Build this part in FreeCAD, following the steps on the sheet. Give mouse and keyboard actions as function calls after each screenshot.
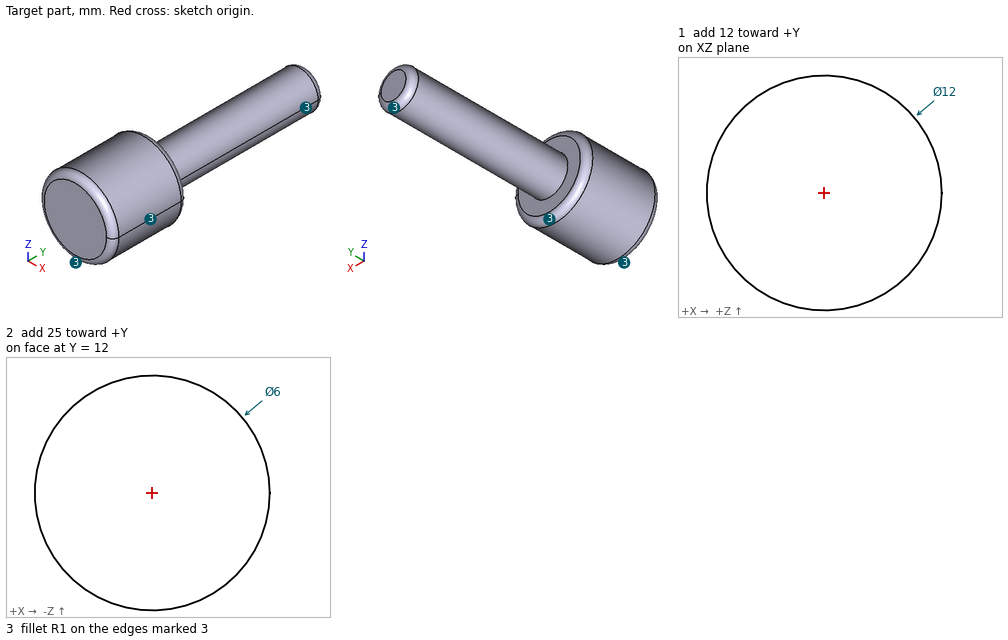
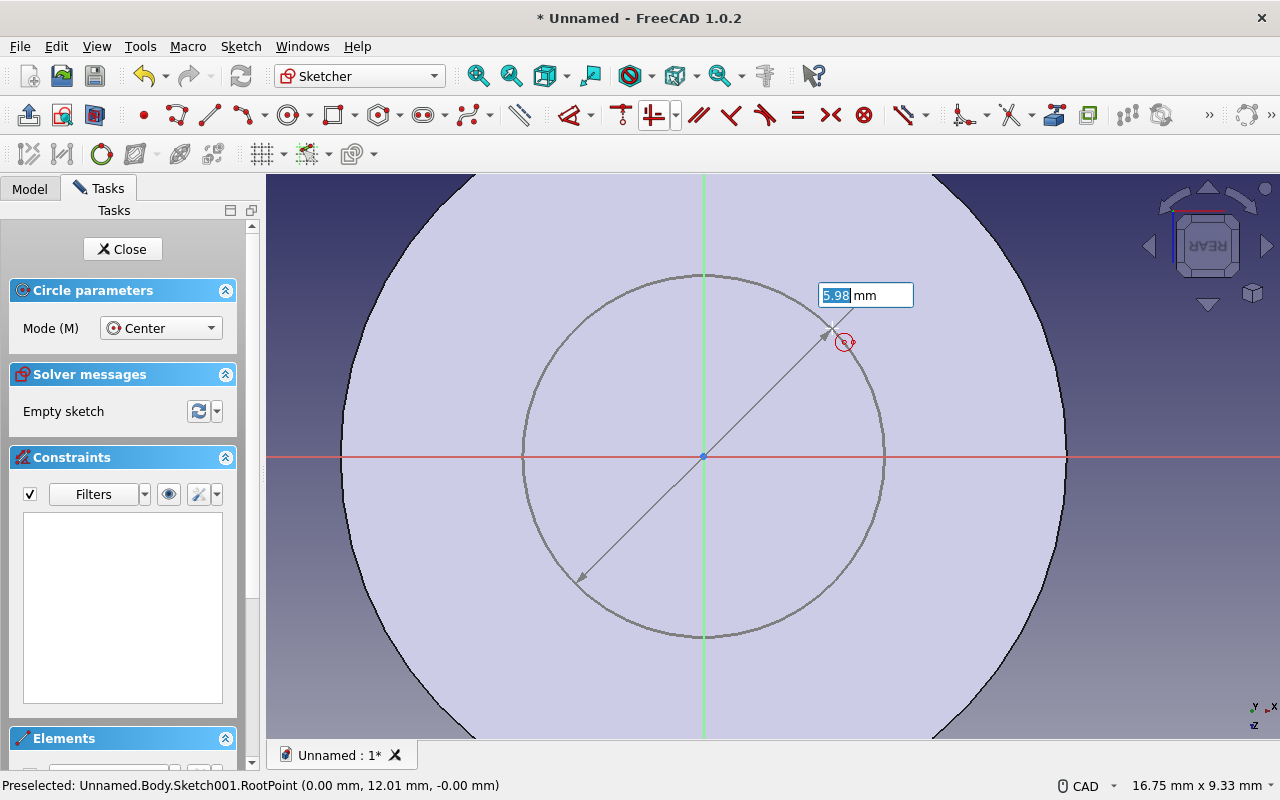
text(6)
key(Return)
key(Escape)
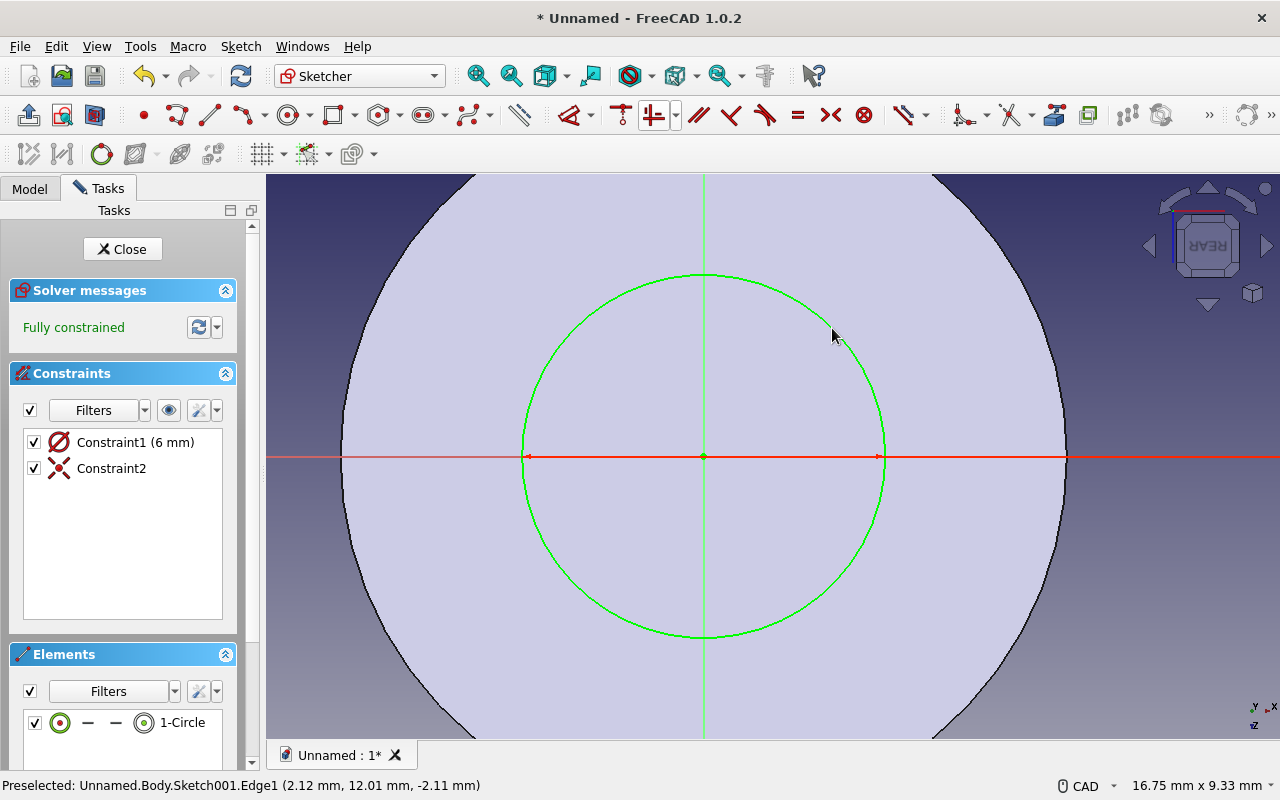
click(123, 249)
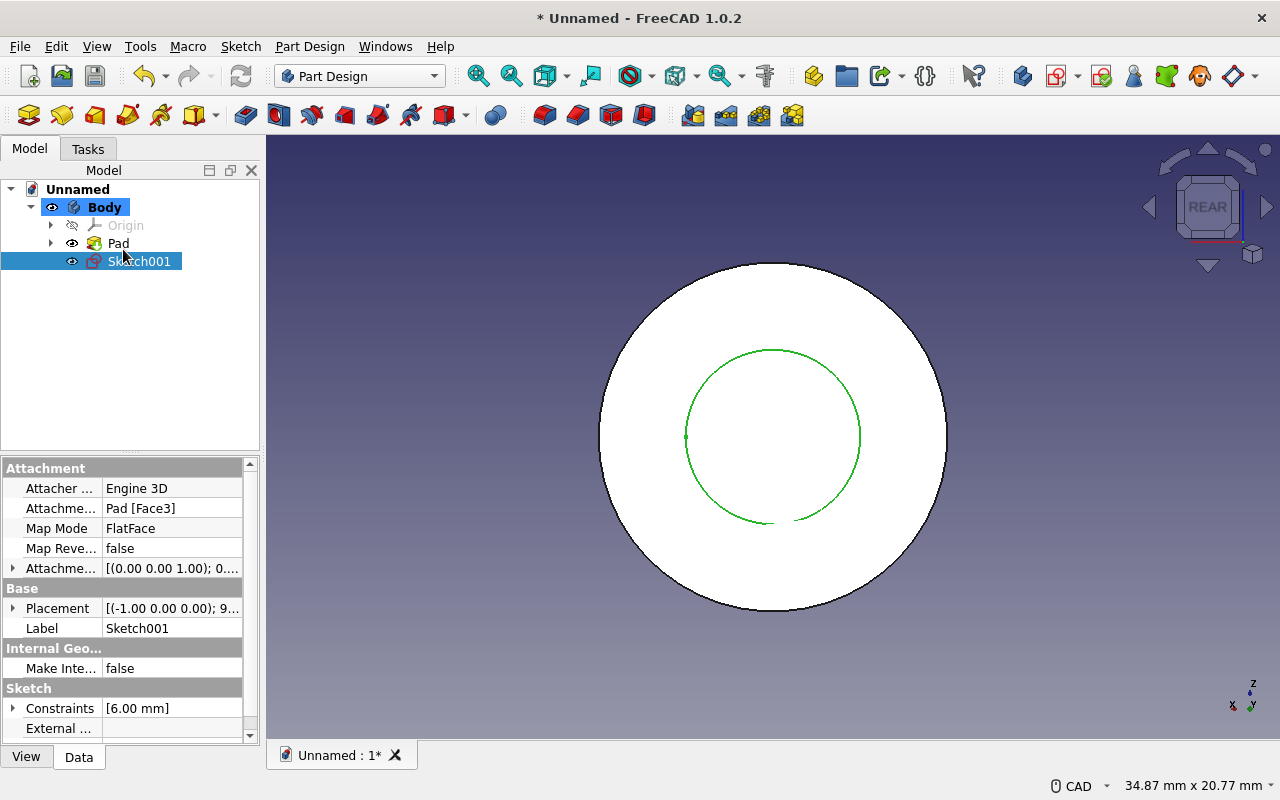
click(29, 116)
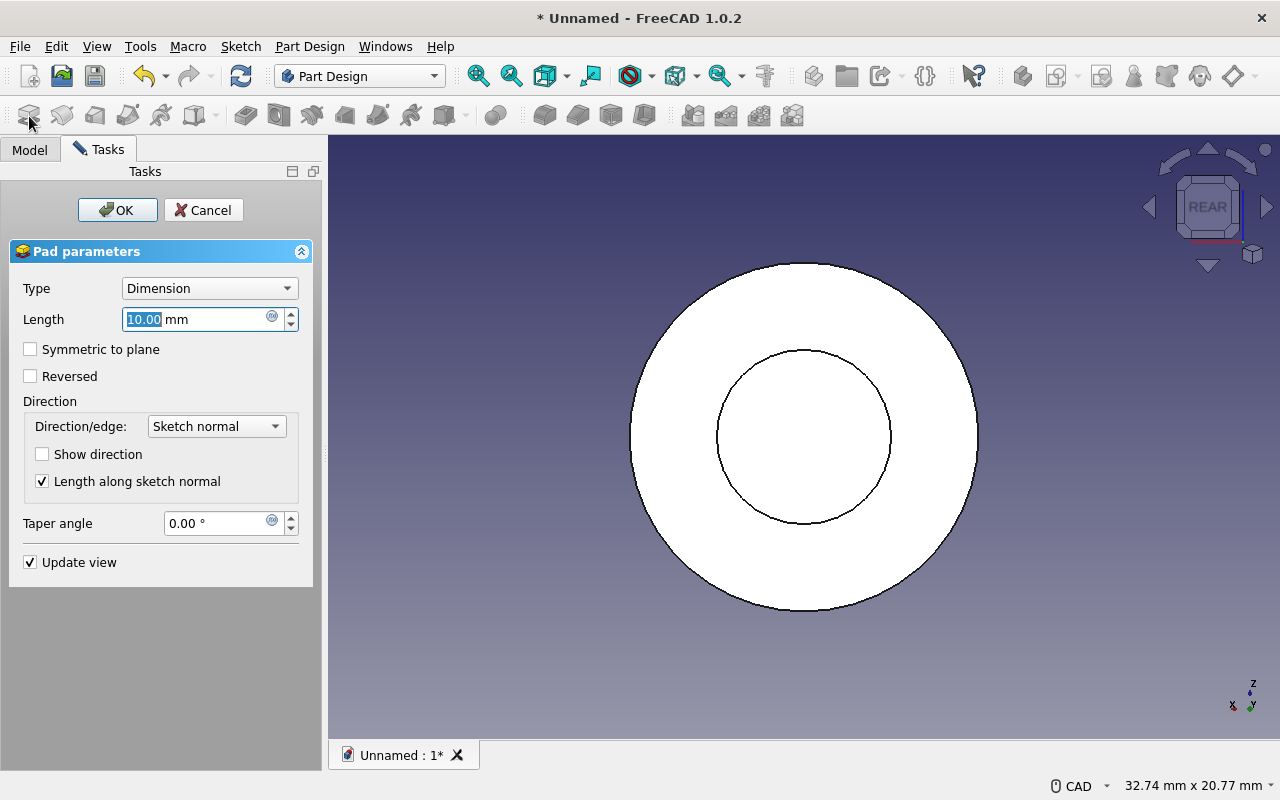
text(25)
key(Tab)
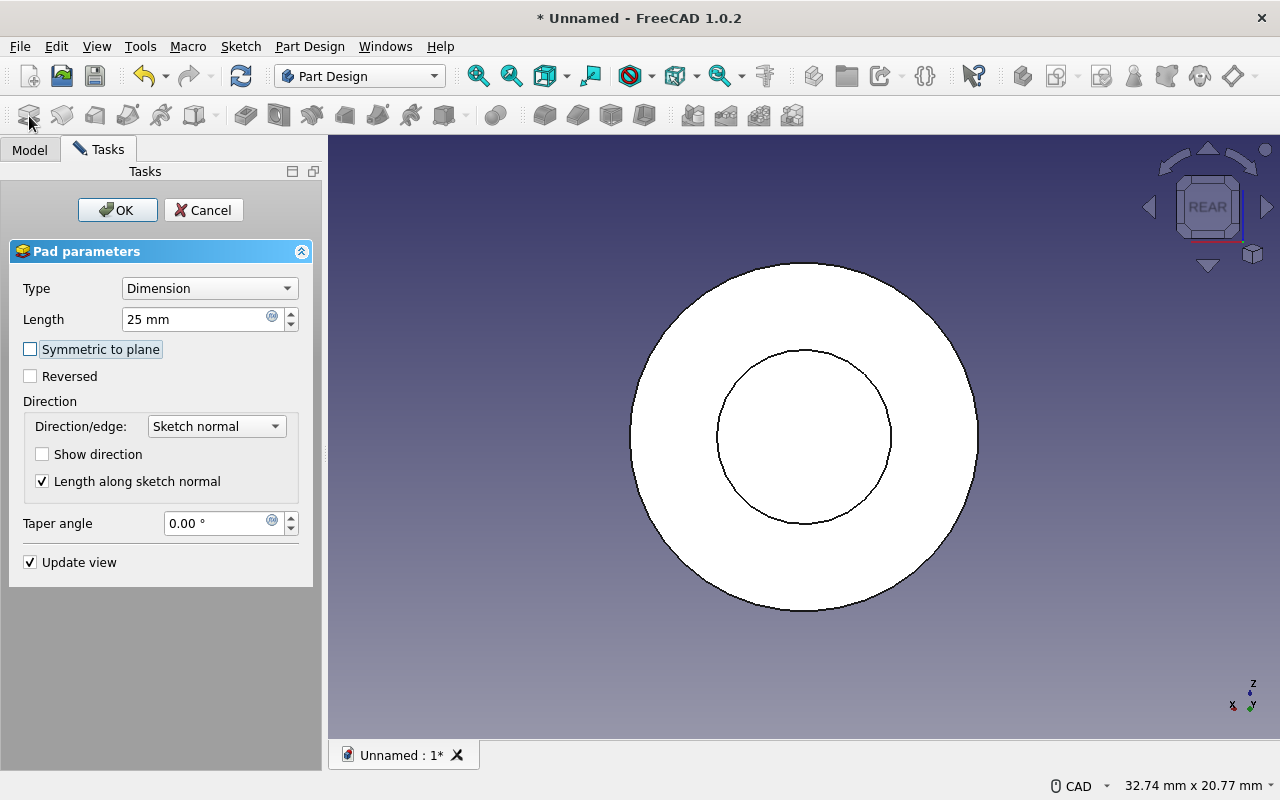
click(118, 210)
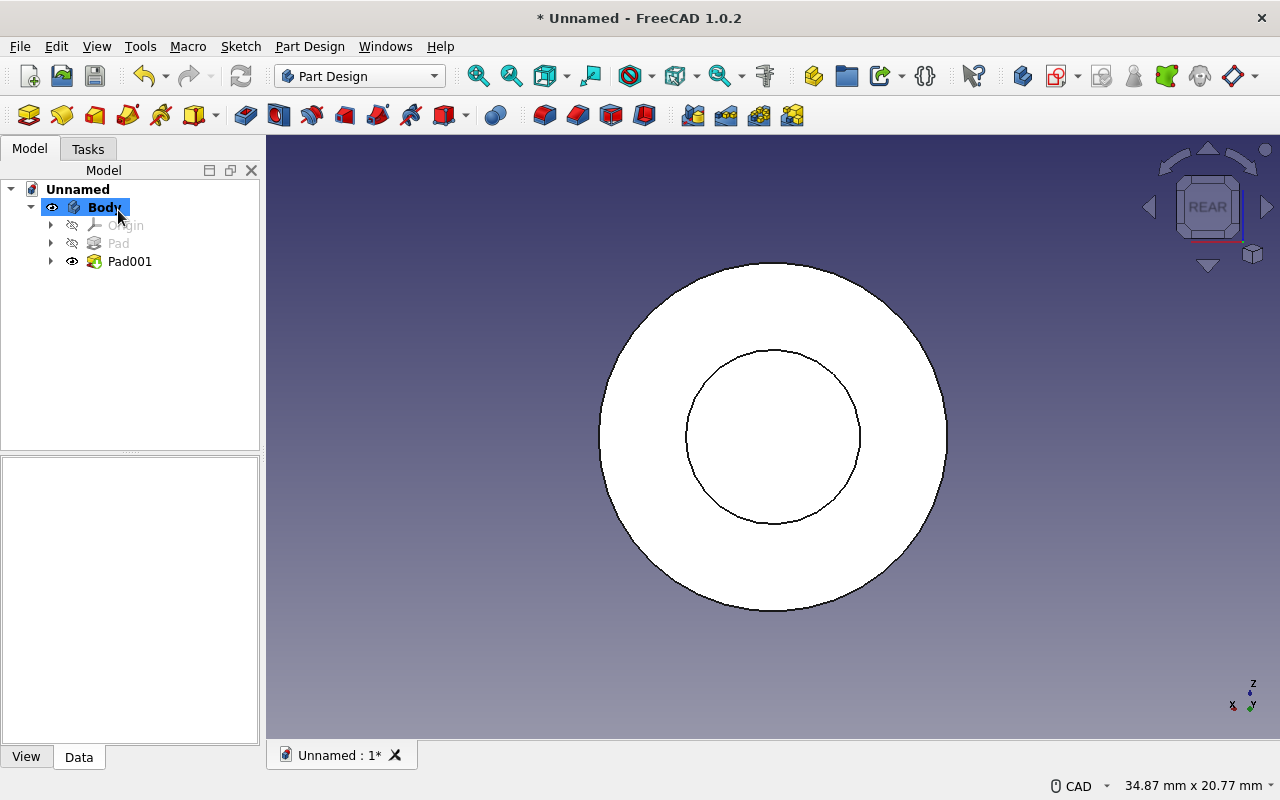
click(947, 436)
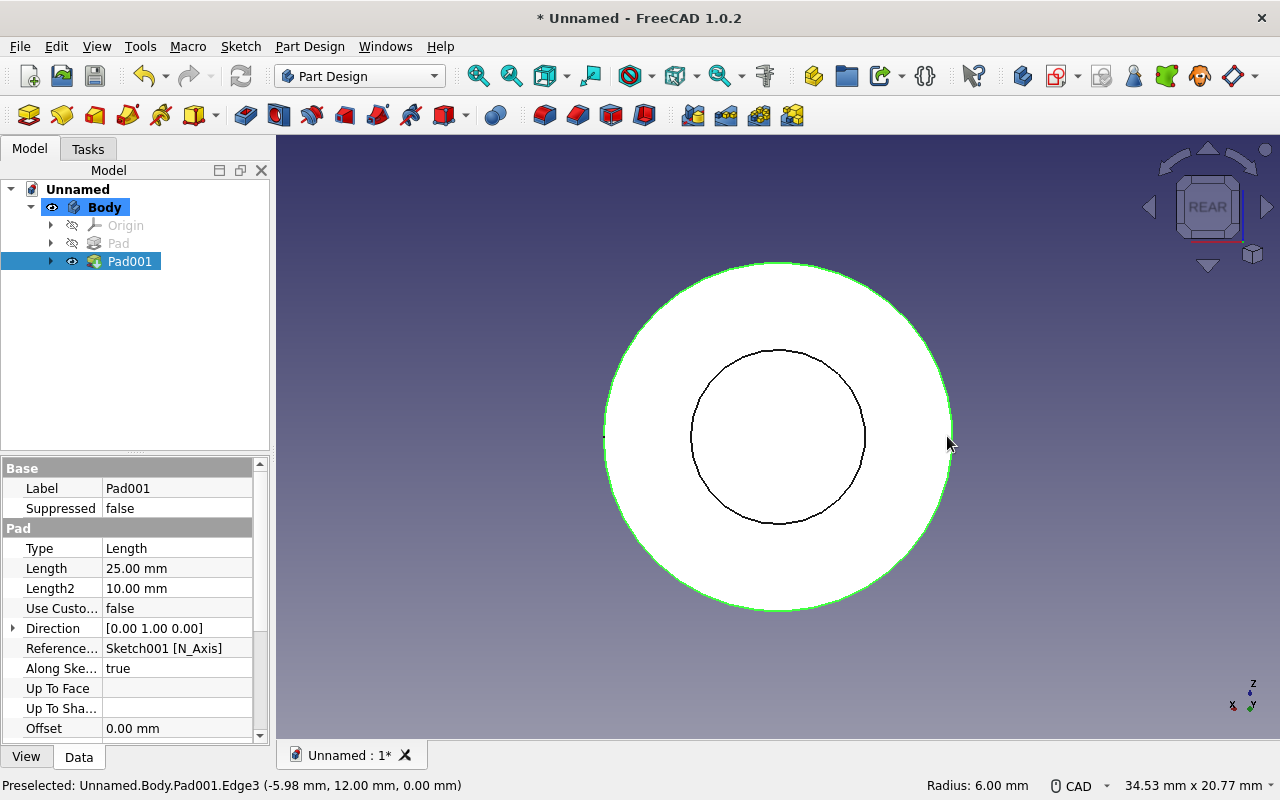
click(865, 436, ctrl)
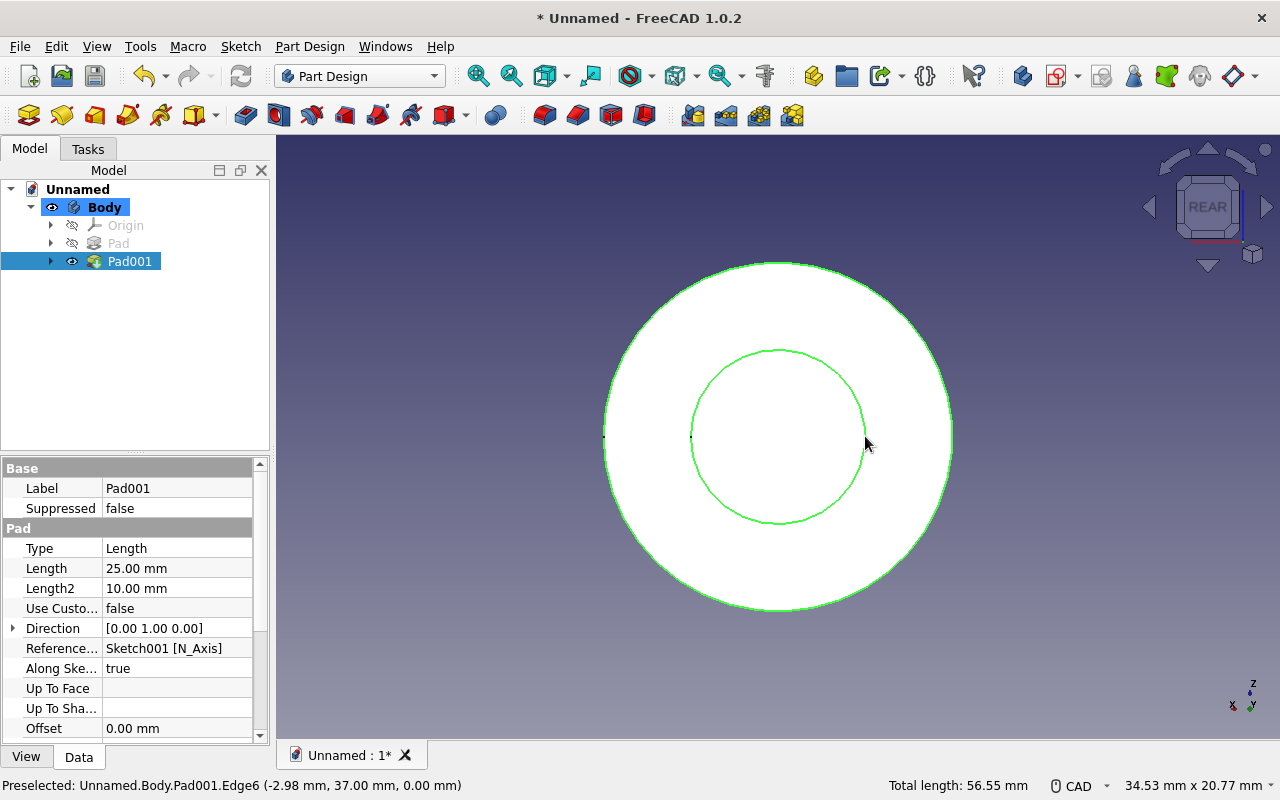
key(0)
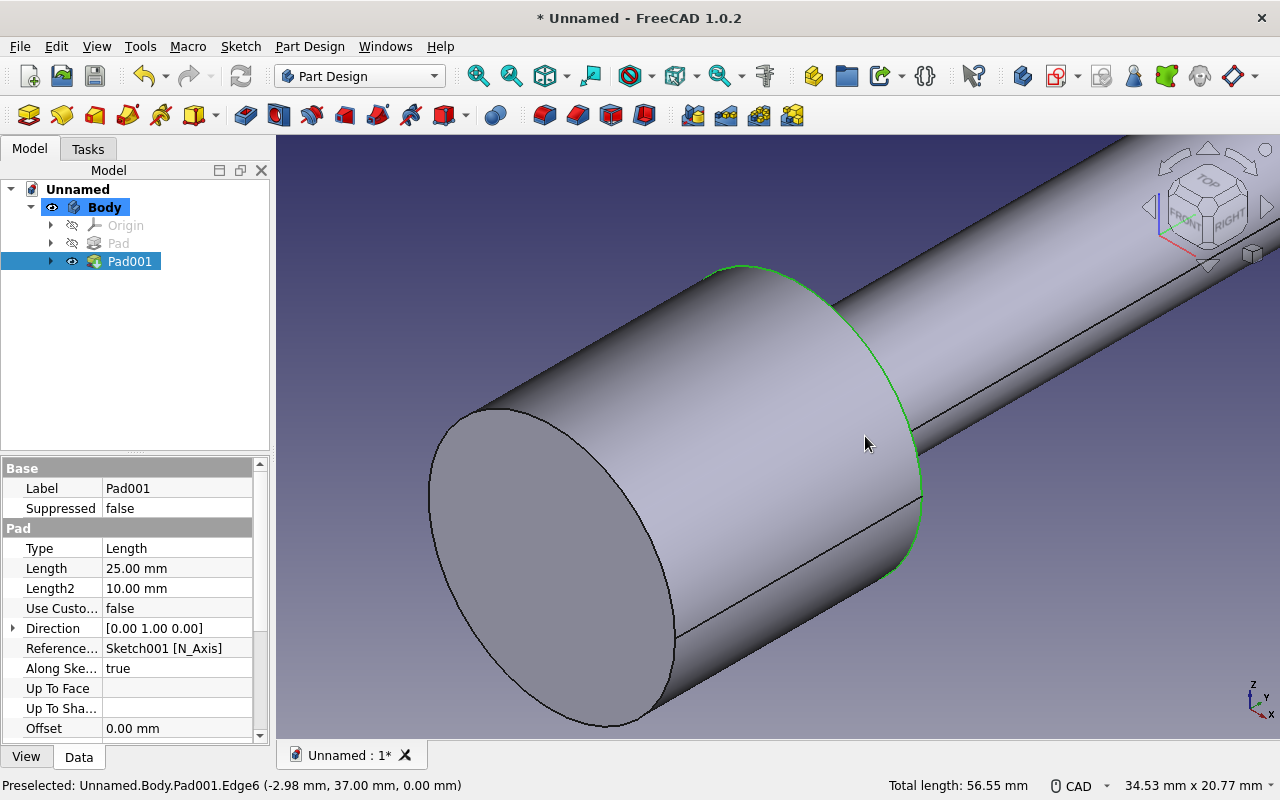
click(479, 76)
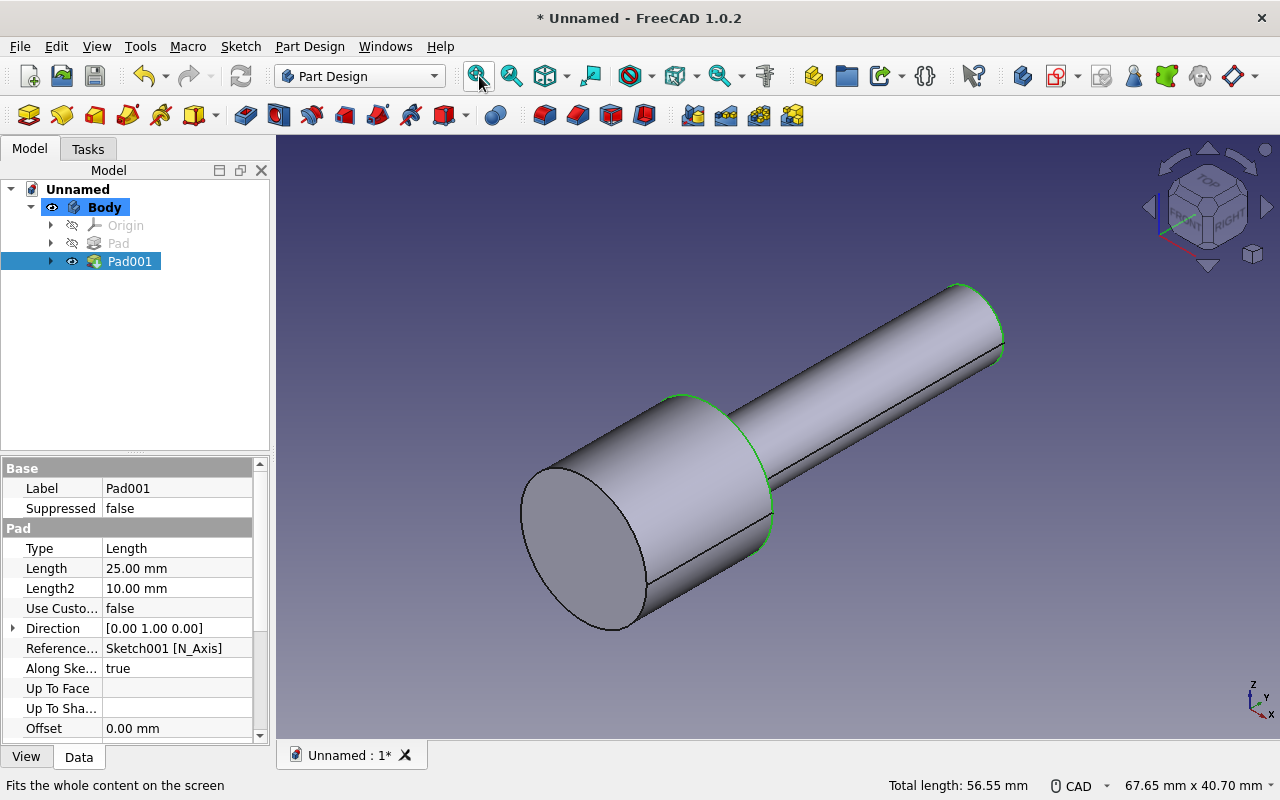
click(564, 468, ctrl)